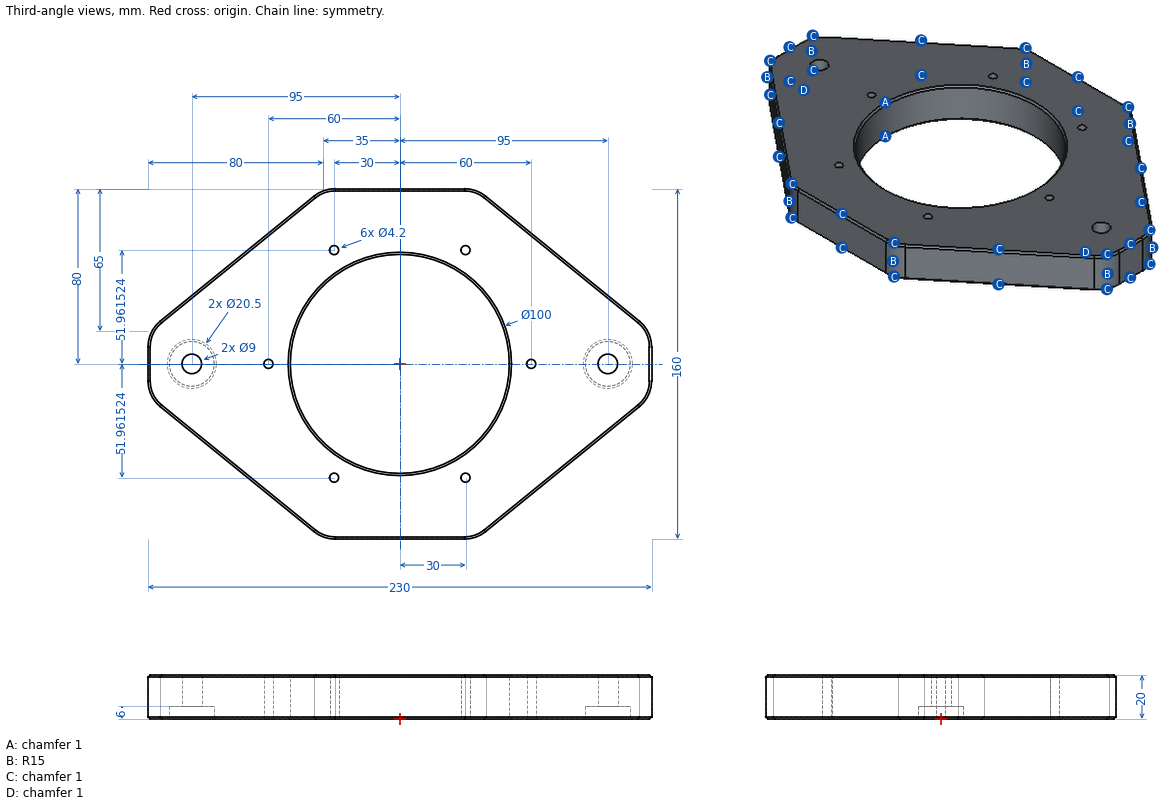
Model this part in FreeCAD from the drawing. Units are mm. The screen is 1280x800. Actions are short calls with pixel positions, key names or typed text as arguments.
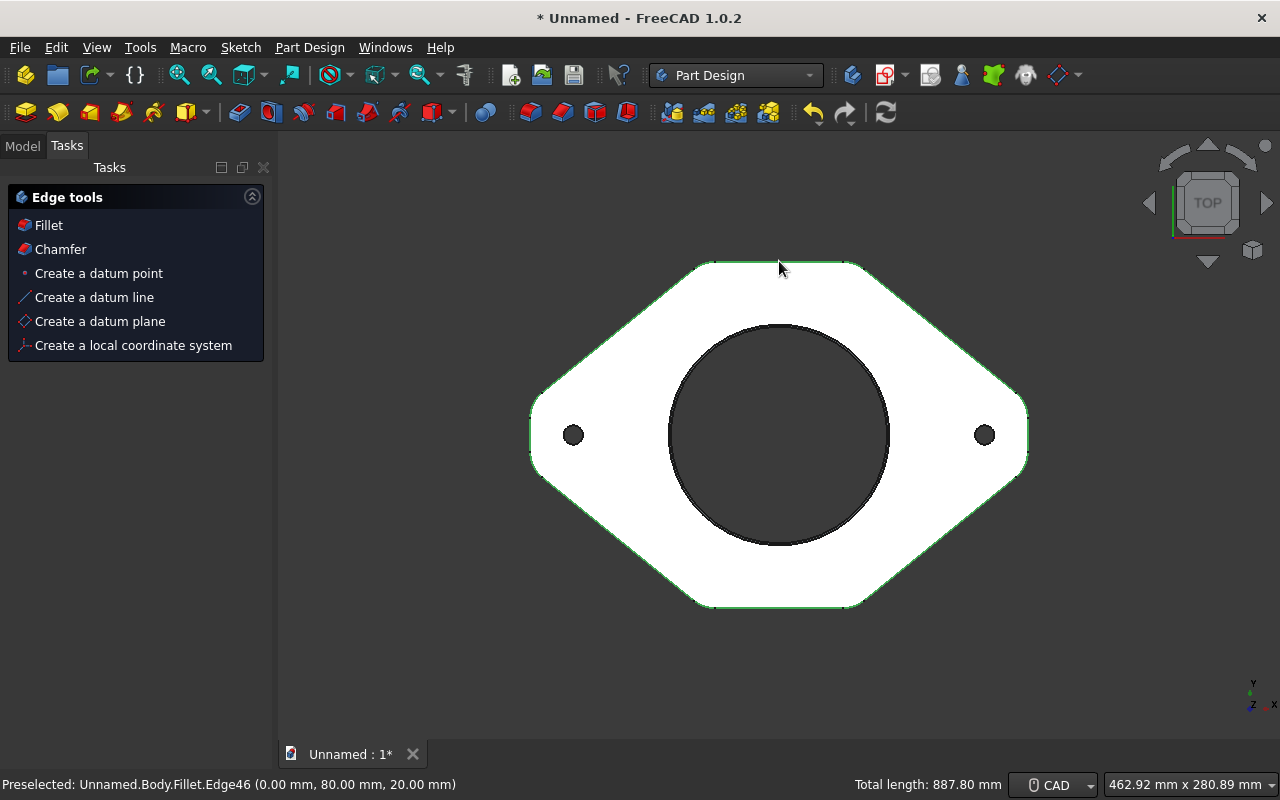
key(1)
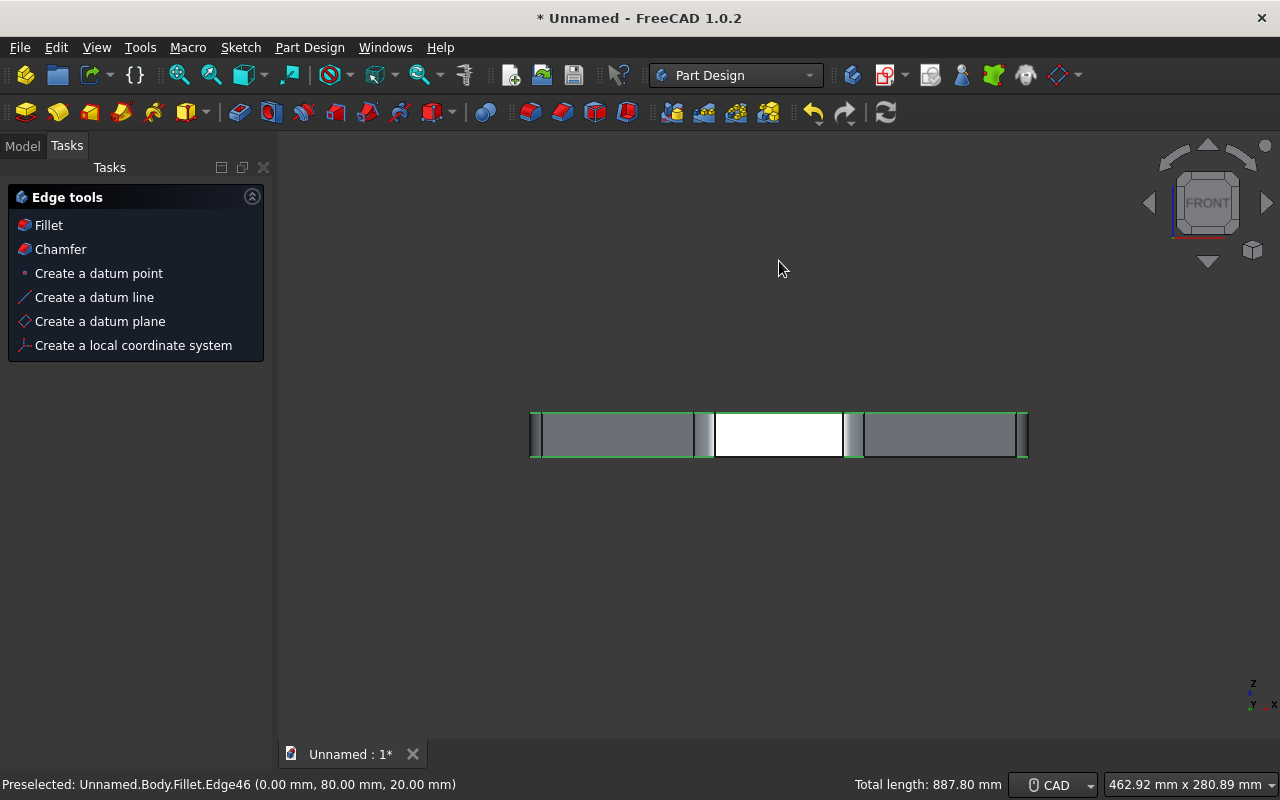
click(940, 456, ctrl)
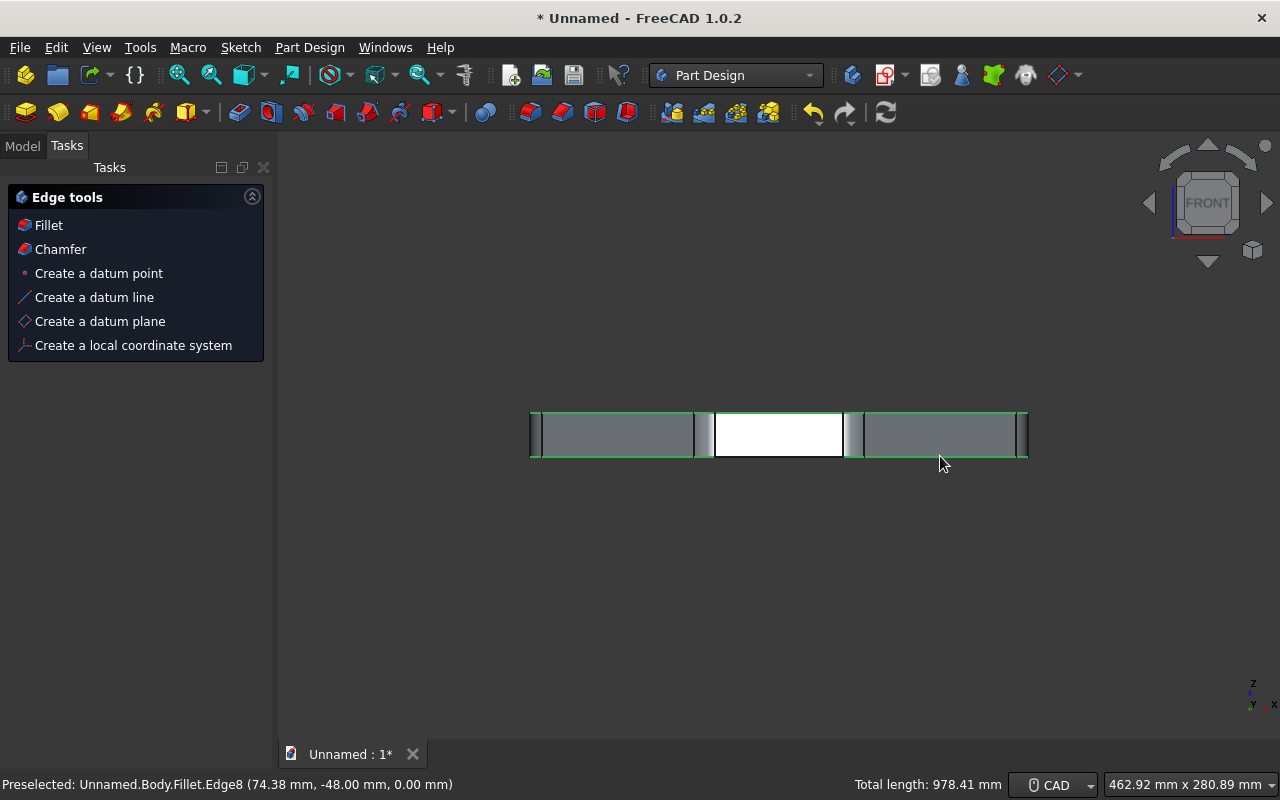
click(779, 456, ctrl)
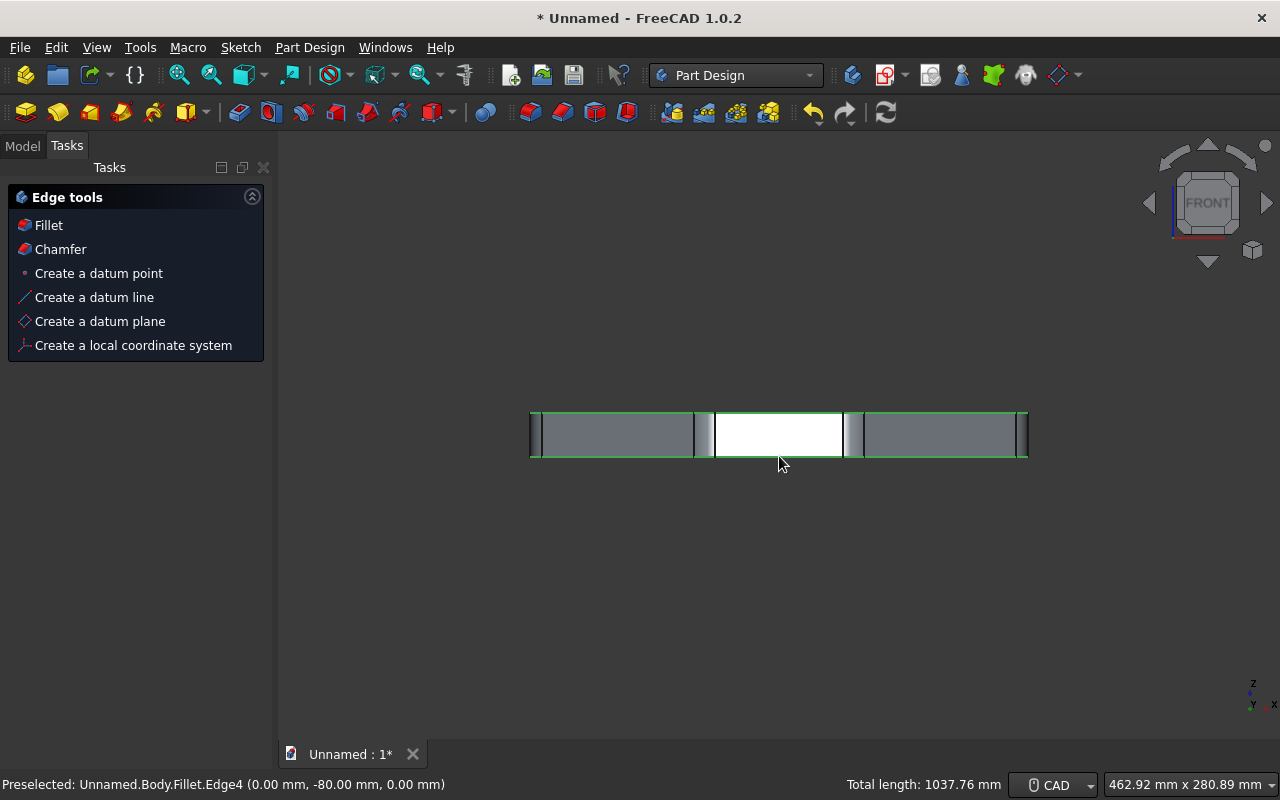
key(3)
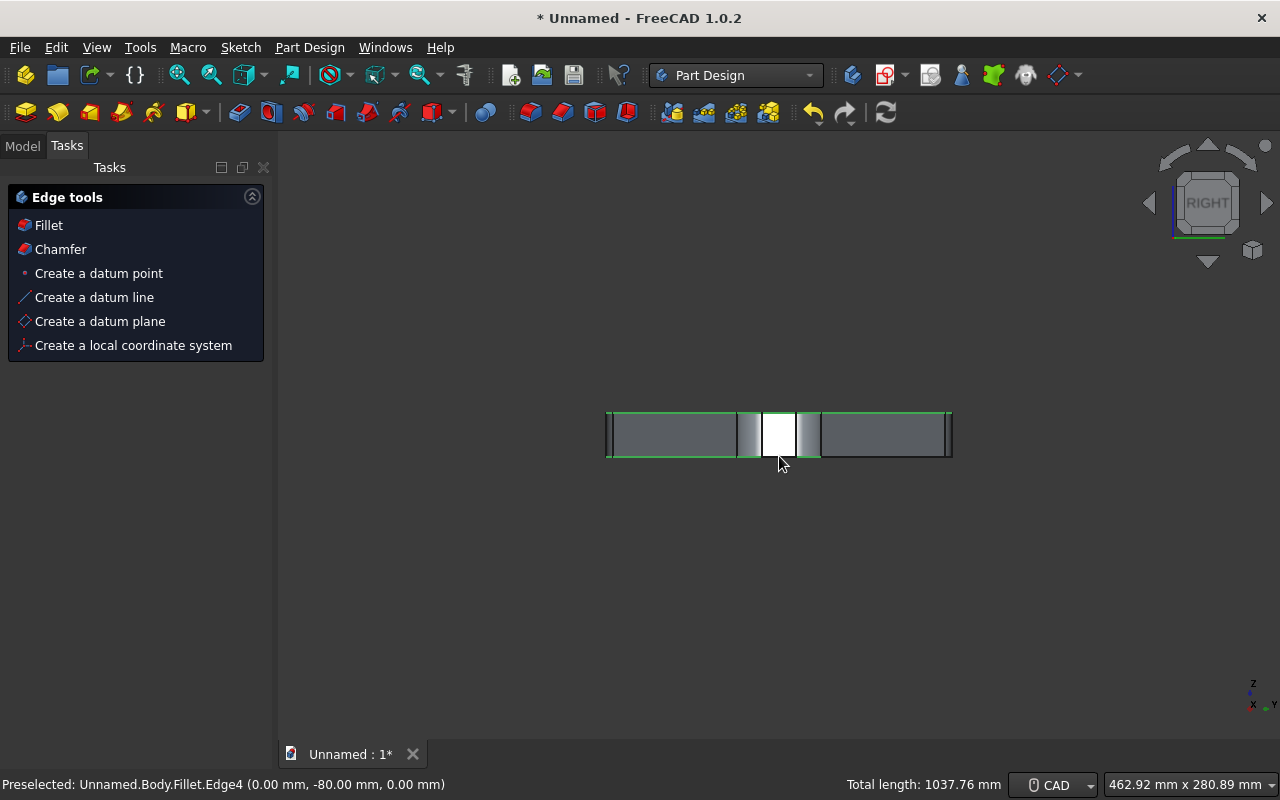
click(180, 76)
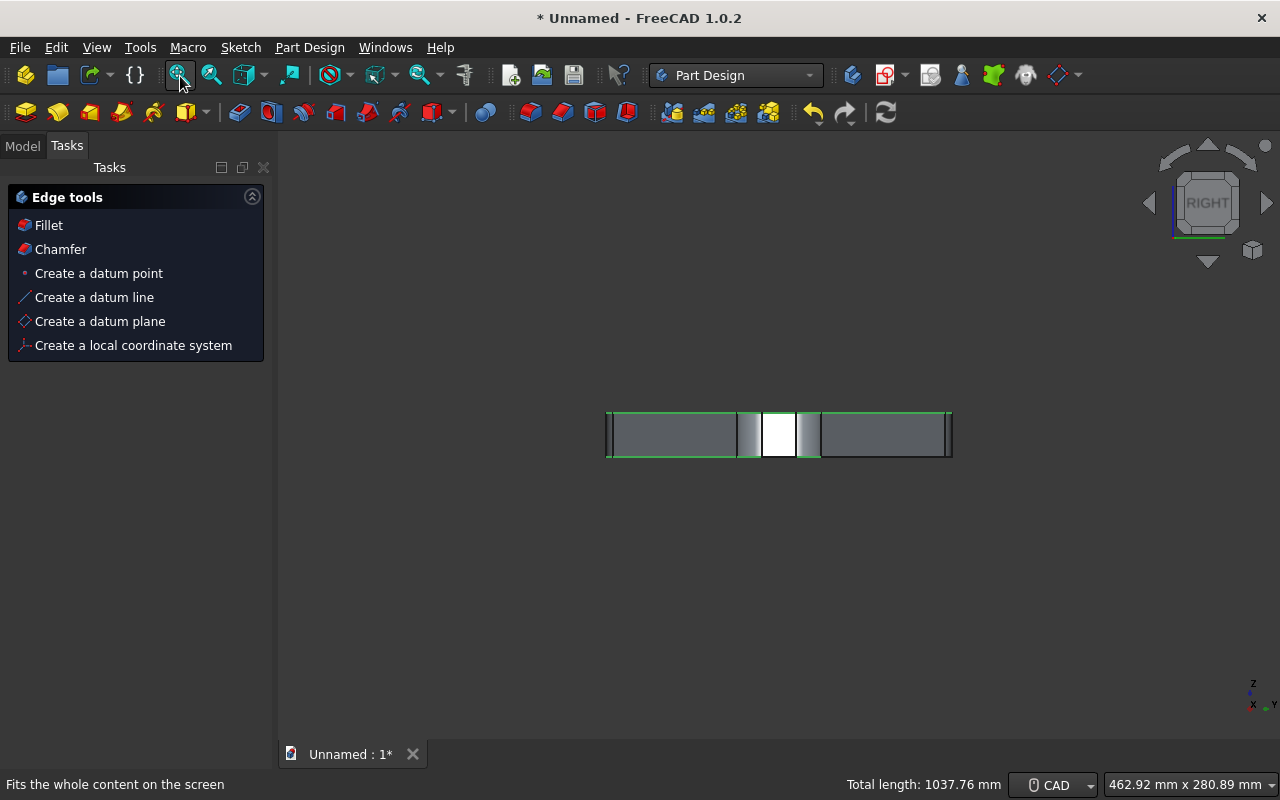
click(883, 456, ctrl)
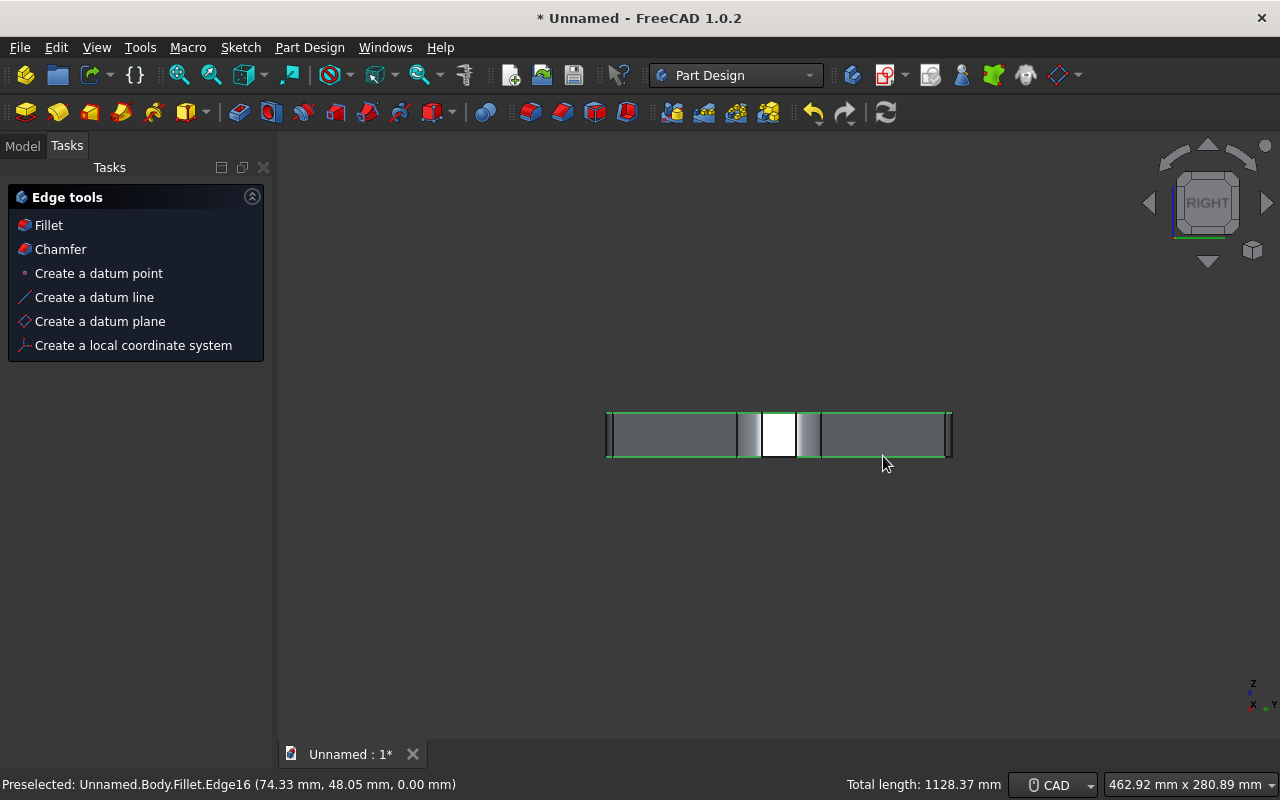
click(779, 456, ctrl)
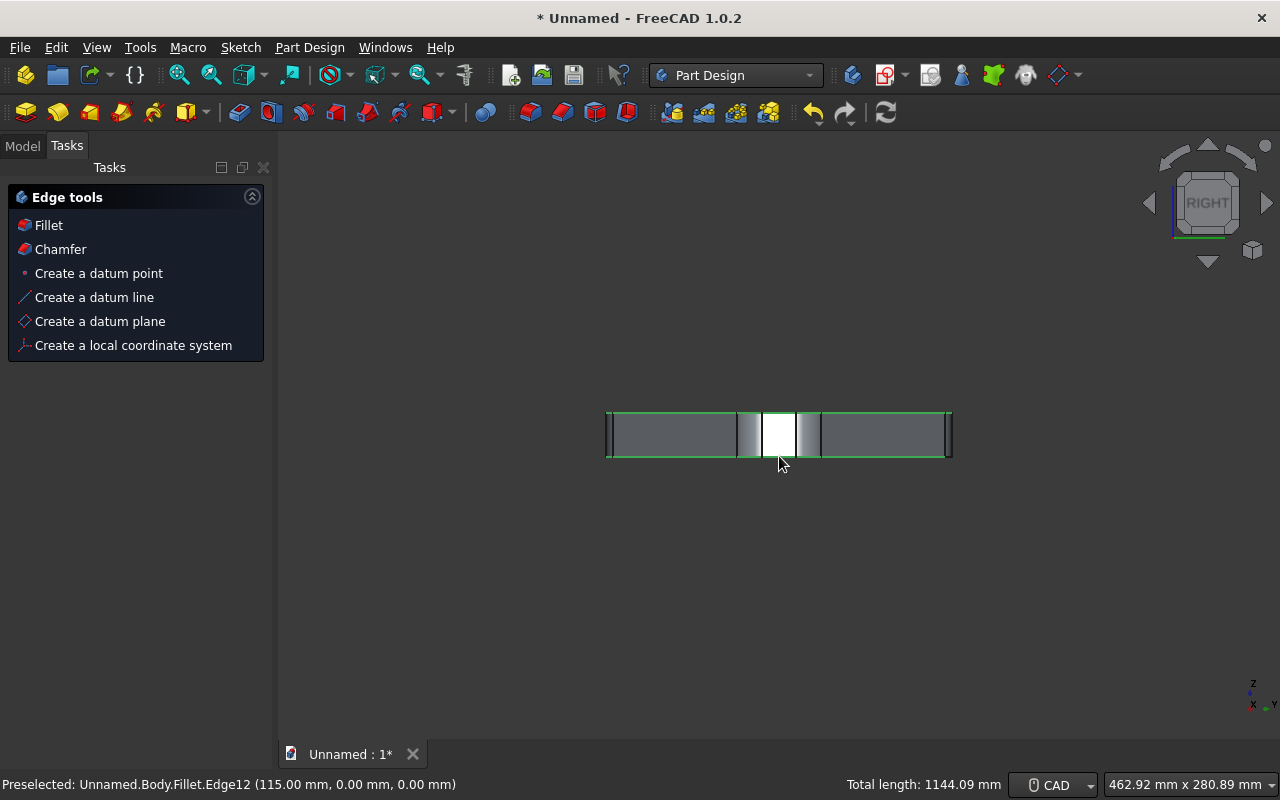
click(951, 456, ctrl)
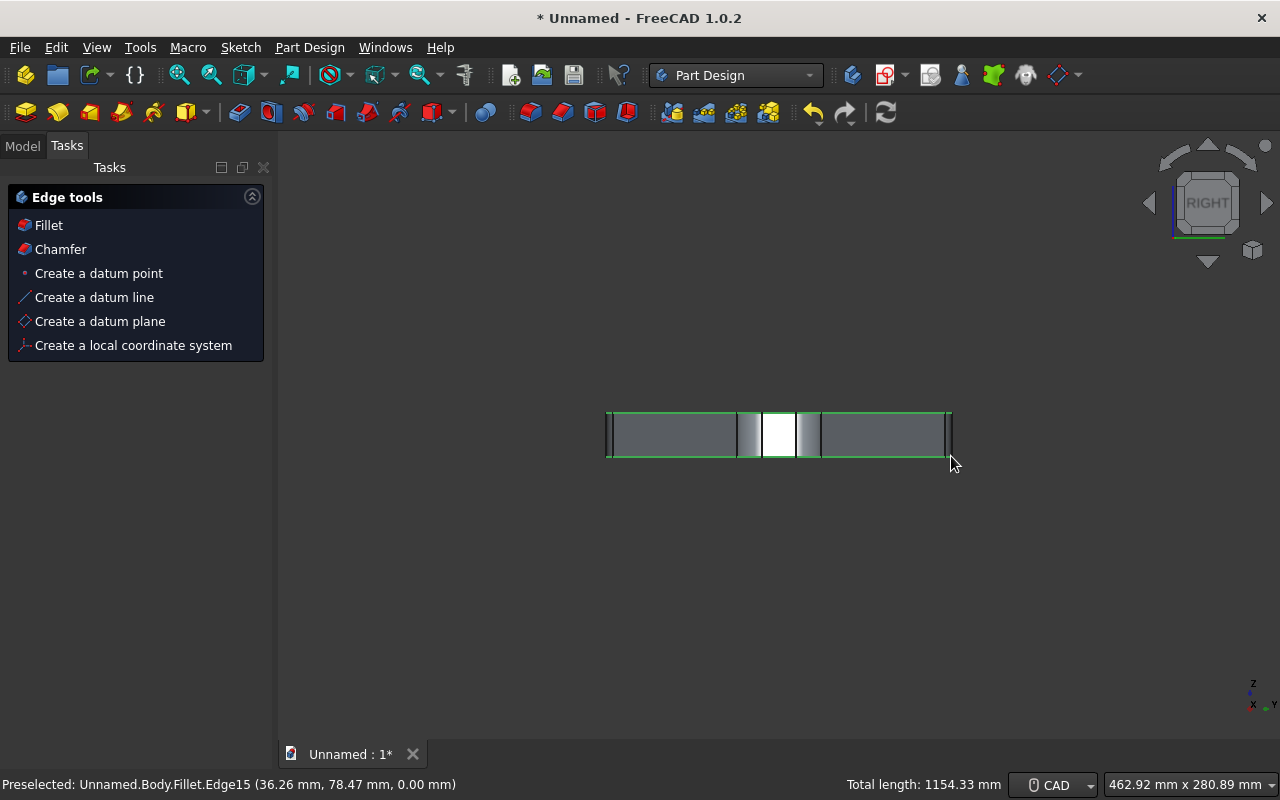
key(5)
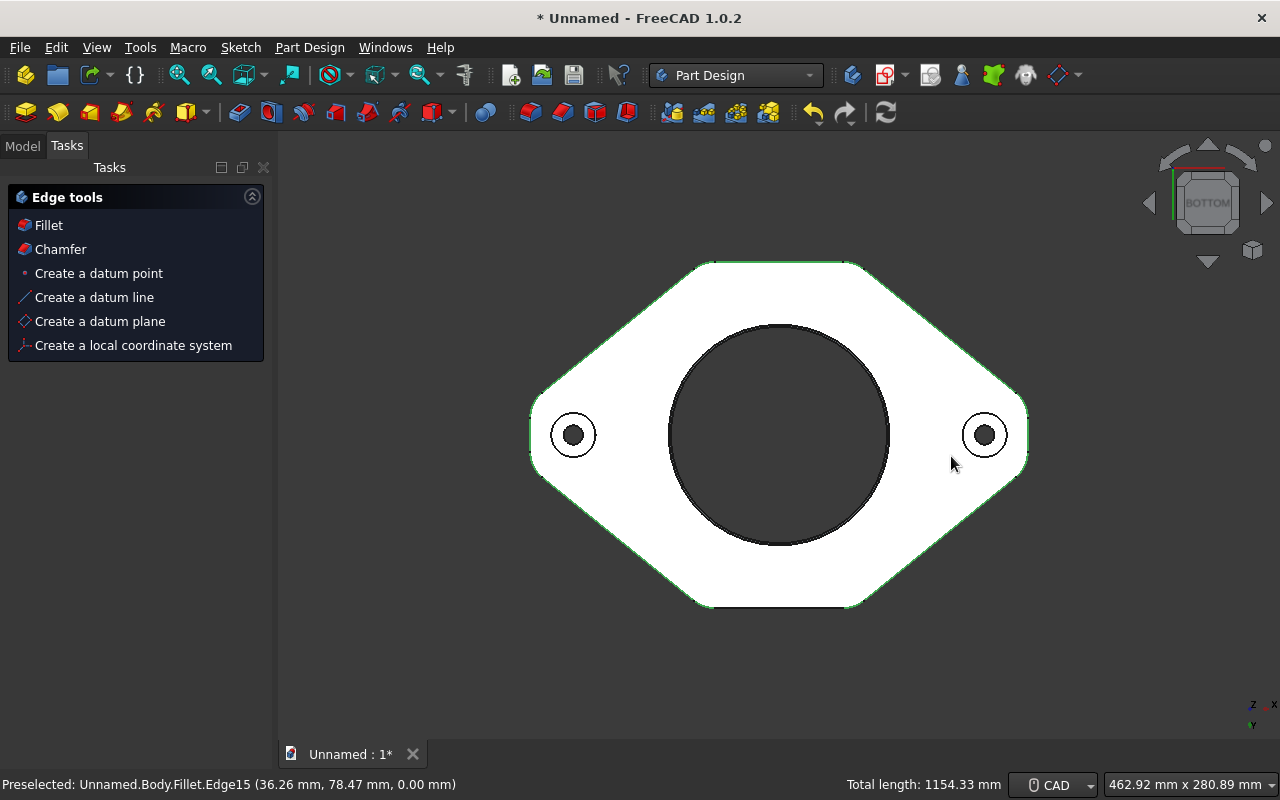
key(4)